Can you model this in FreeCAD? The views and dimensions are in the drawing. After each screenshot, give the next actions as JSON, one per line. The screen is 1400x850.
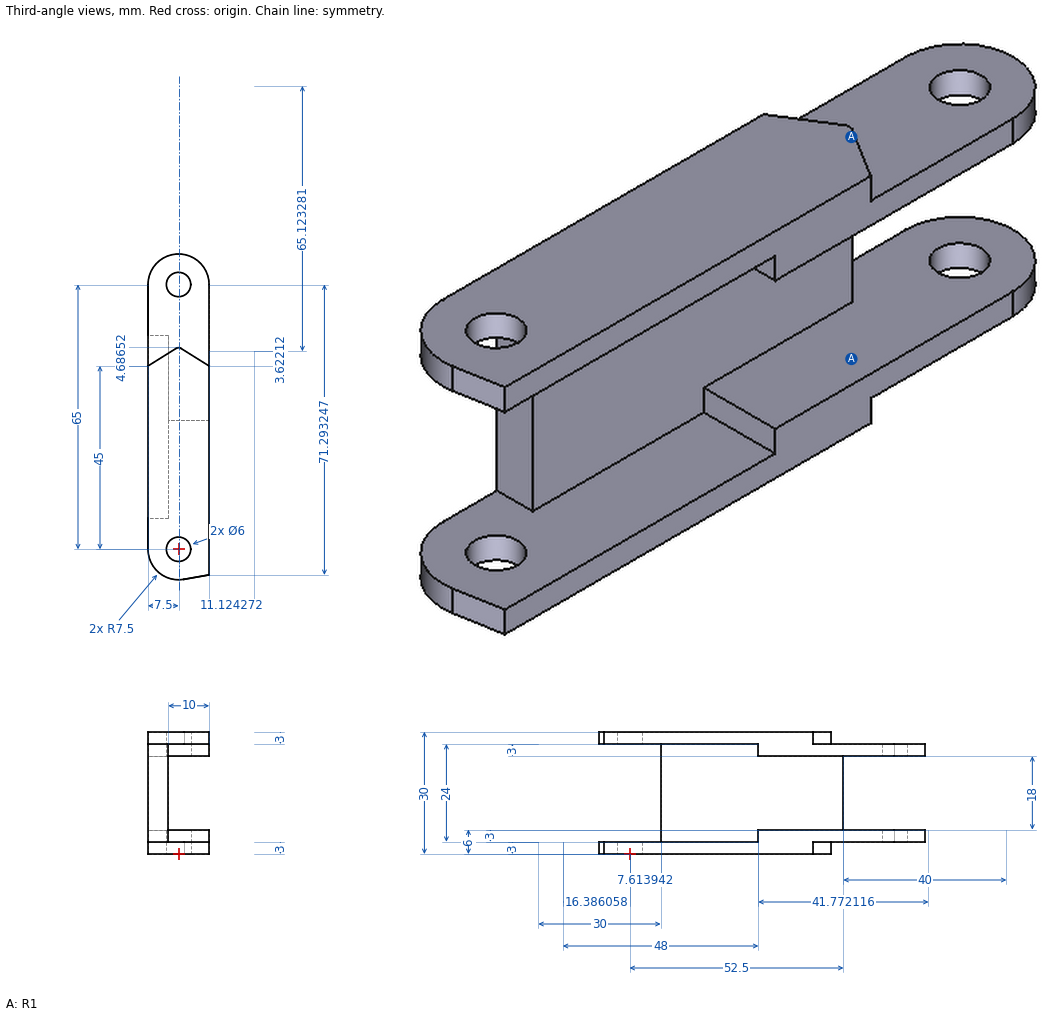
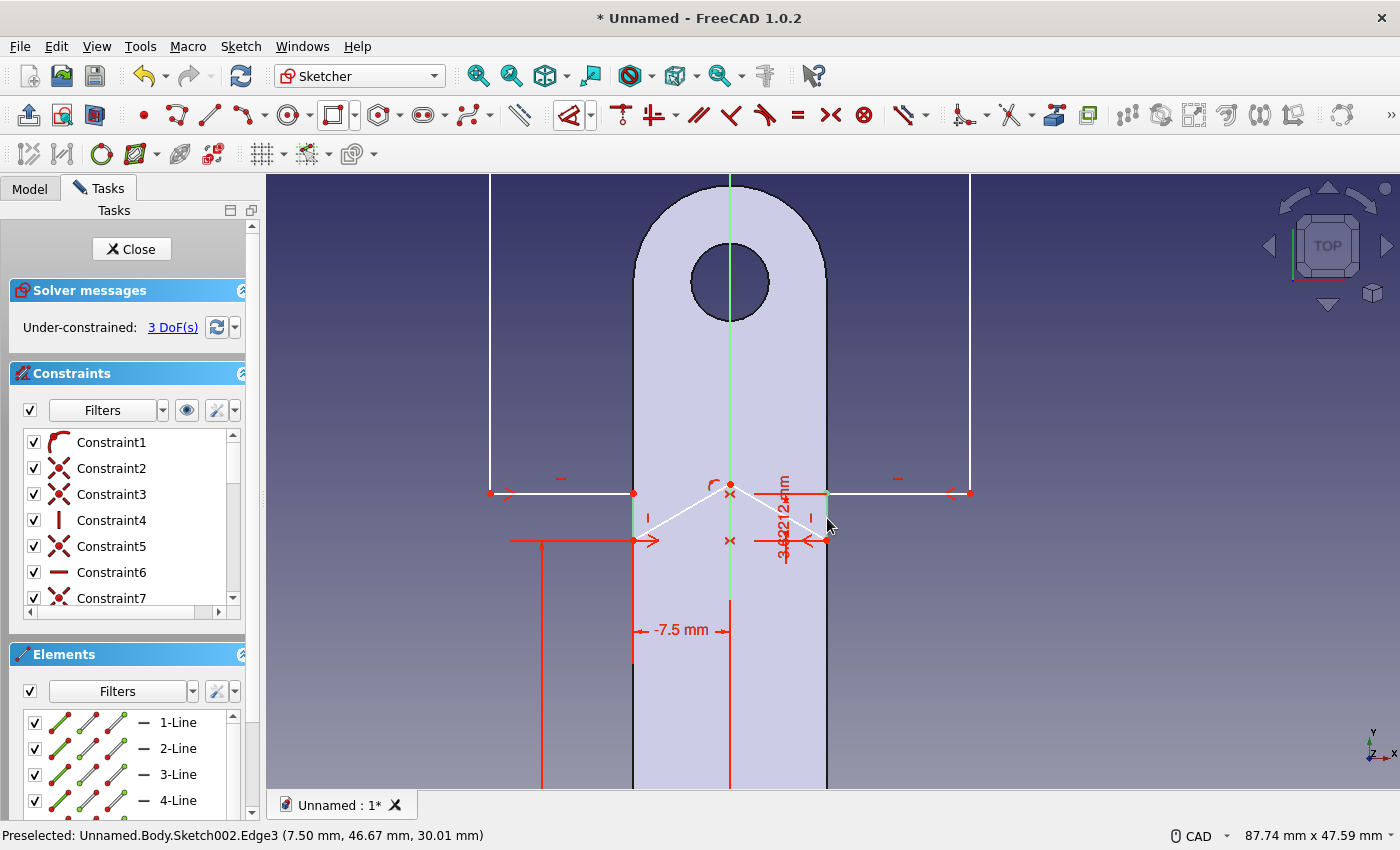
{"action": "left_click", "coordinate": [662, 524]}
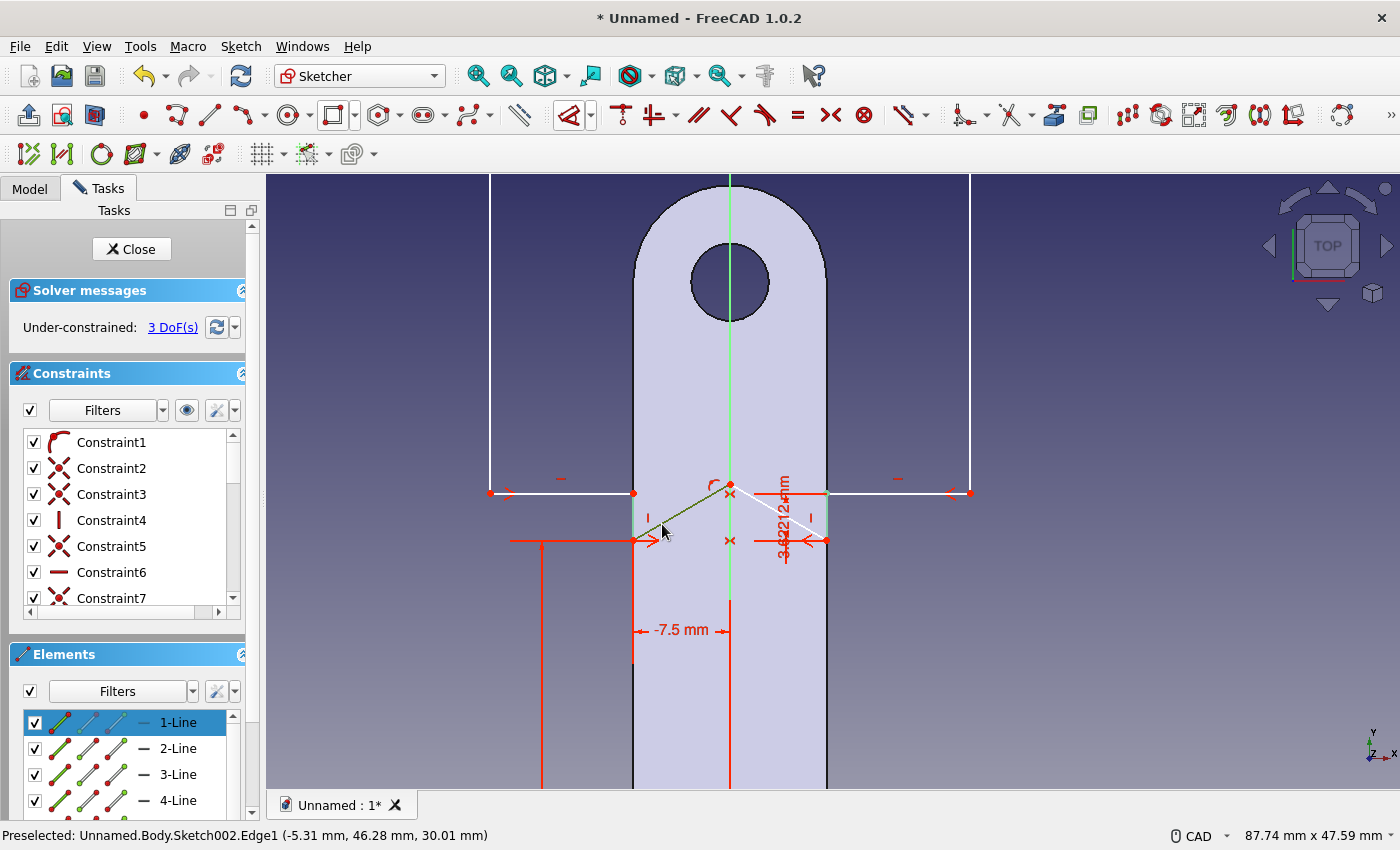
{"action": "key", "text": "i"}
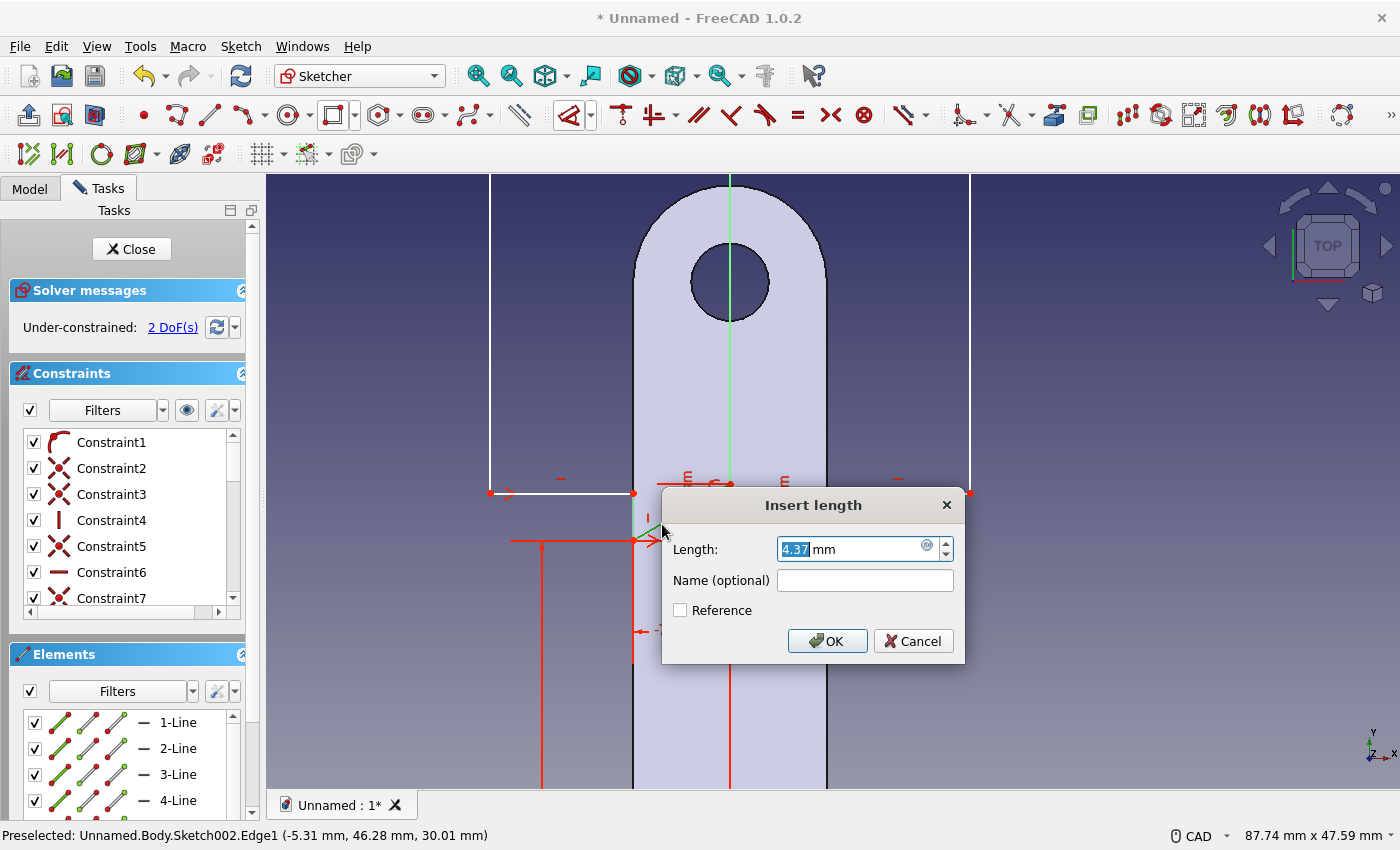
{"action": "type", "text": "4.68652"}
{"action": "key", "text": "Return"}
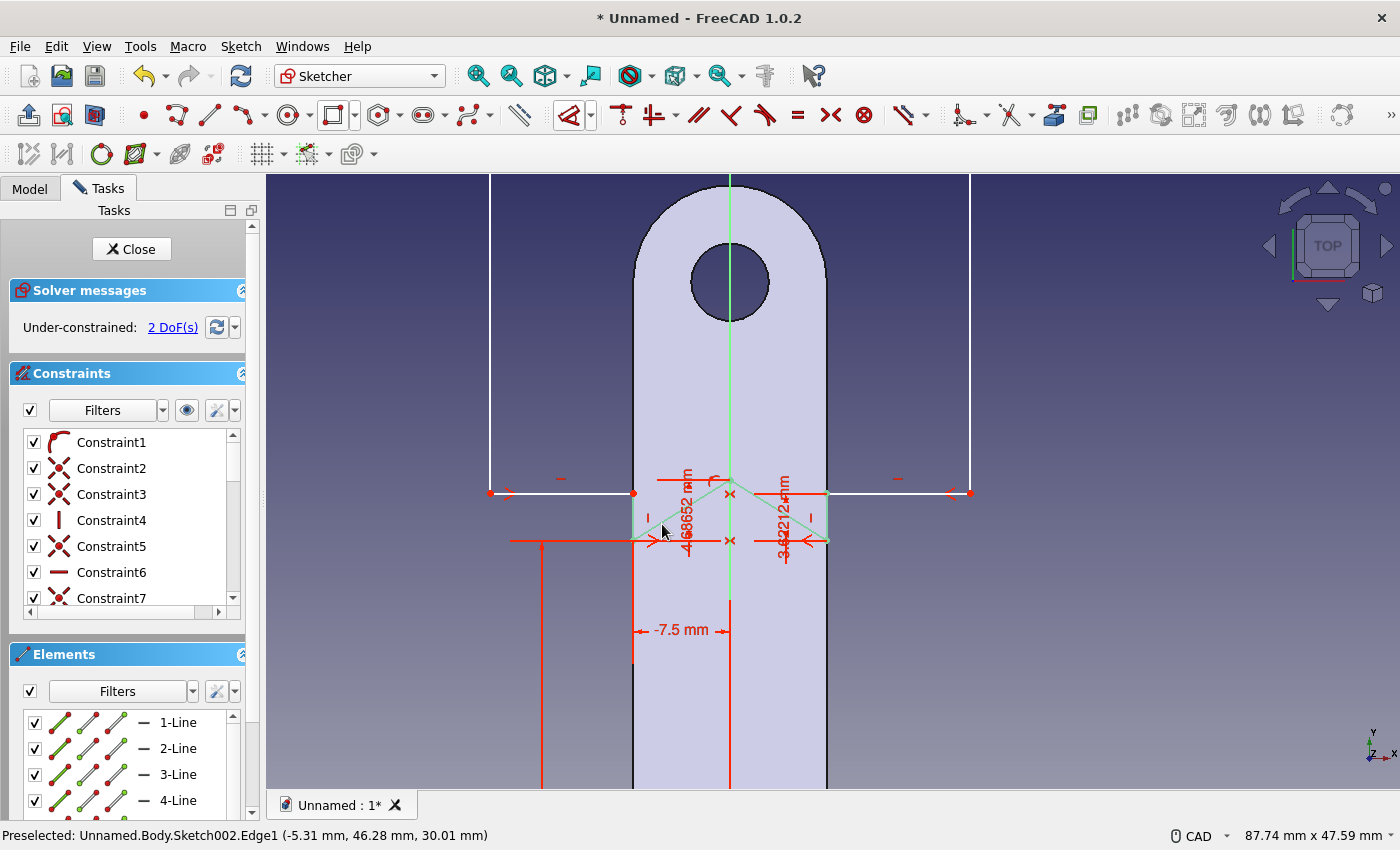
{"action": "scroll", "coordinate": [776, 512], "scroll_direction": "down", "scroll_amount": 7}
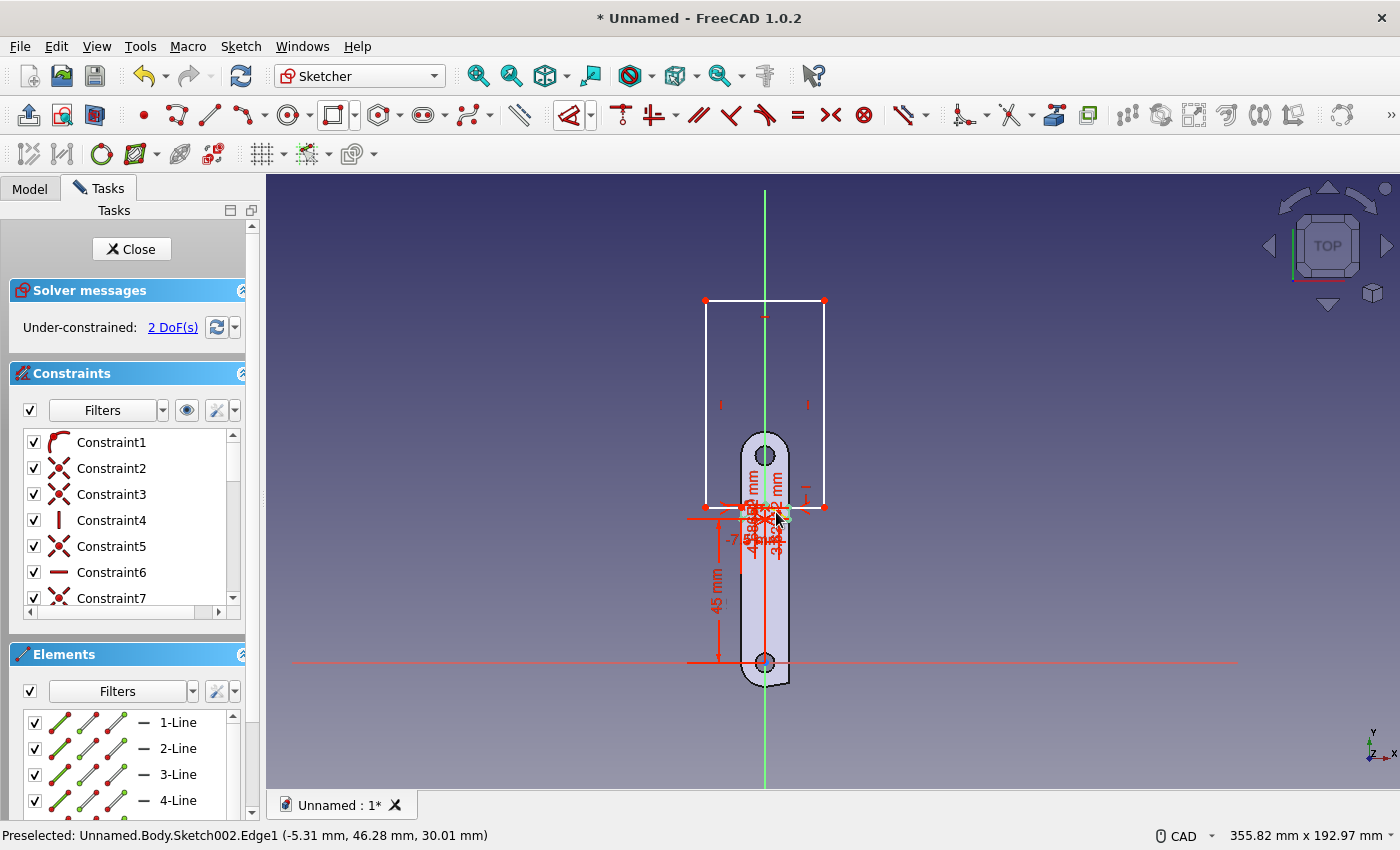
{"action": "scroll", "coordinate": [799, 508], "scroll_direction": "up", "scroll_amount": 2}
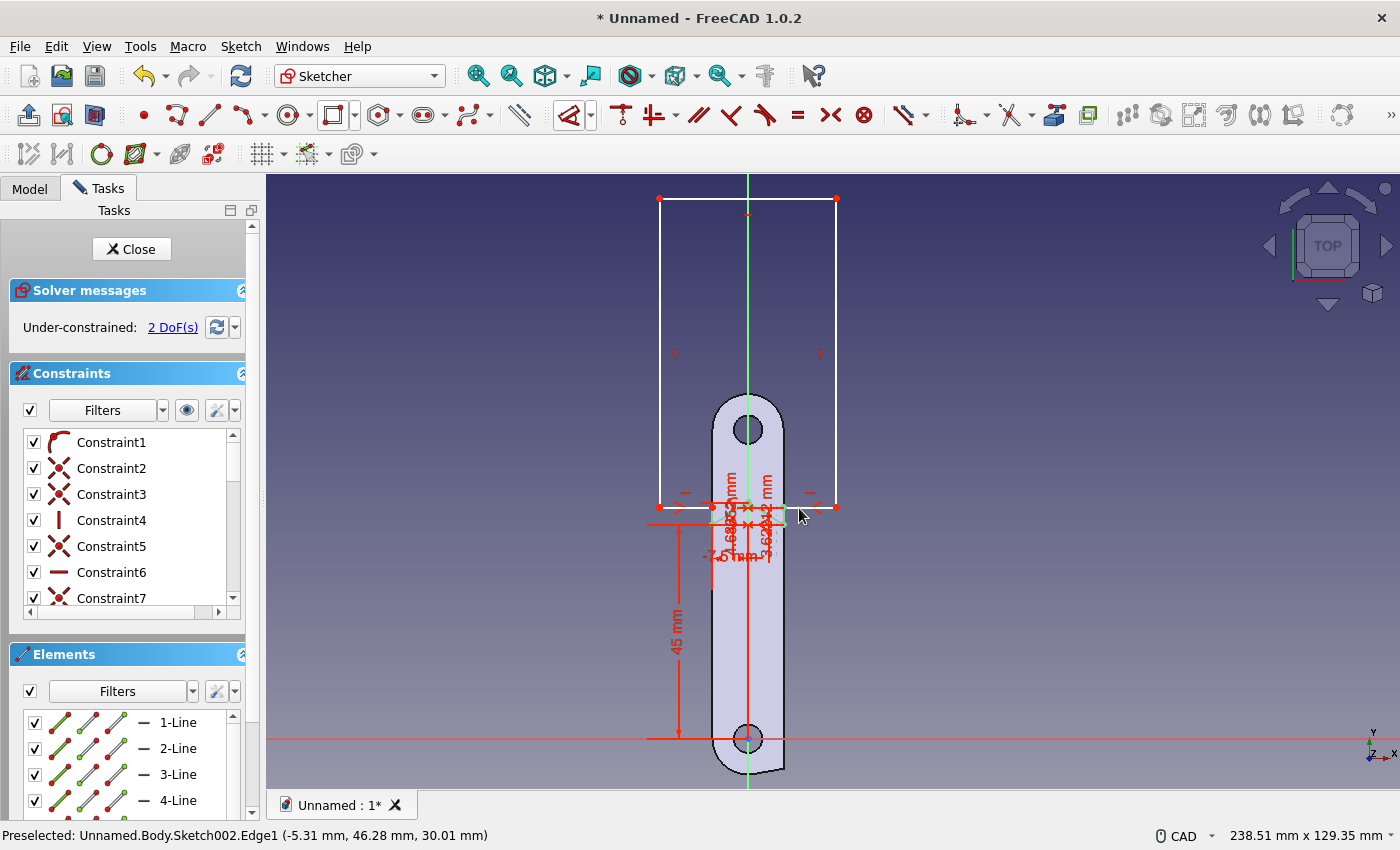
{"action": "left_click", "coordinate": [800, 508]}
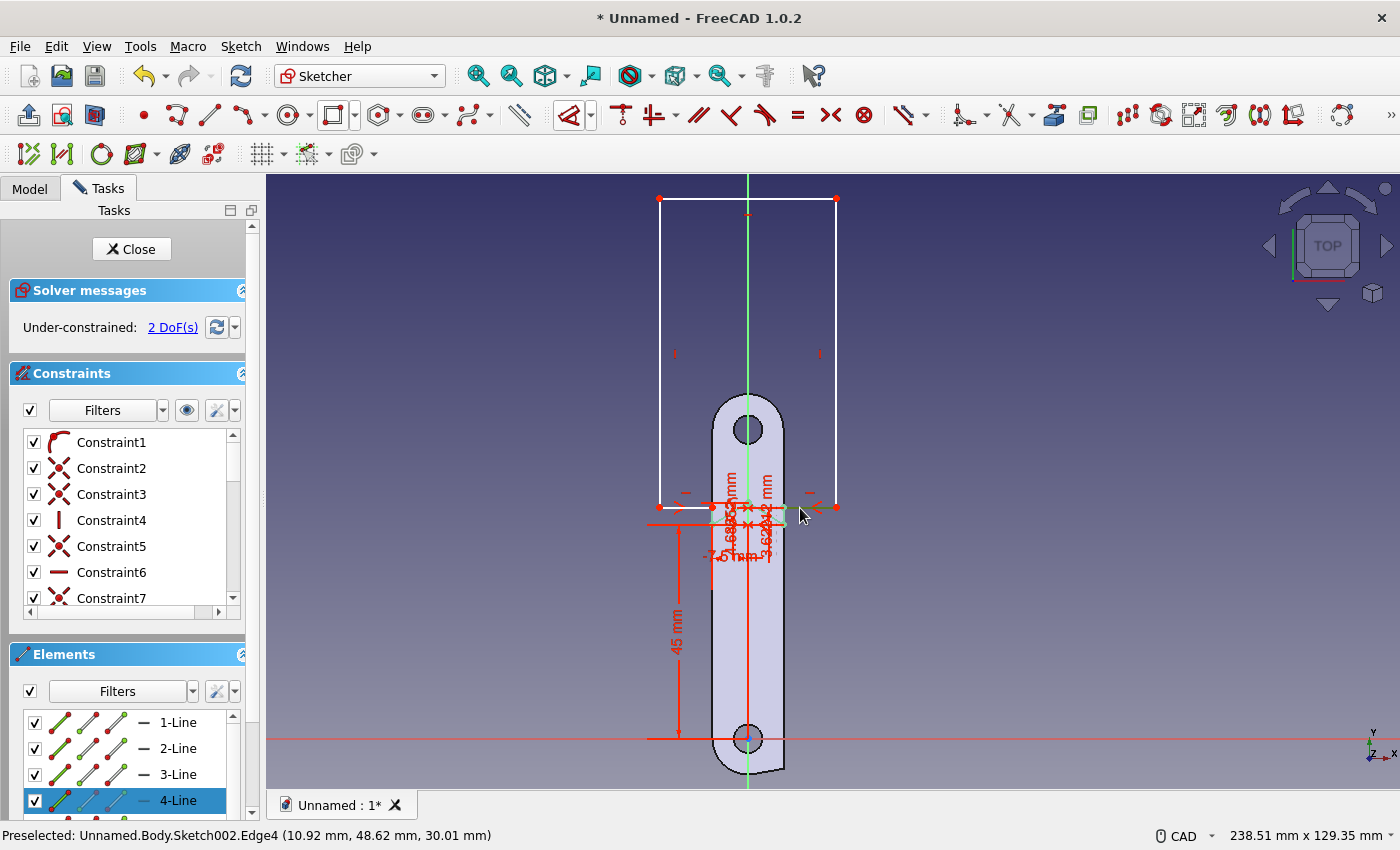
{"action": "key", "text": "l"}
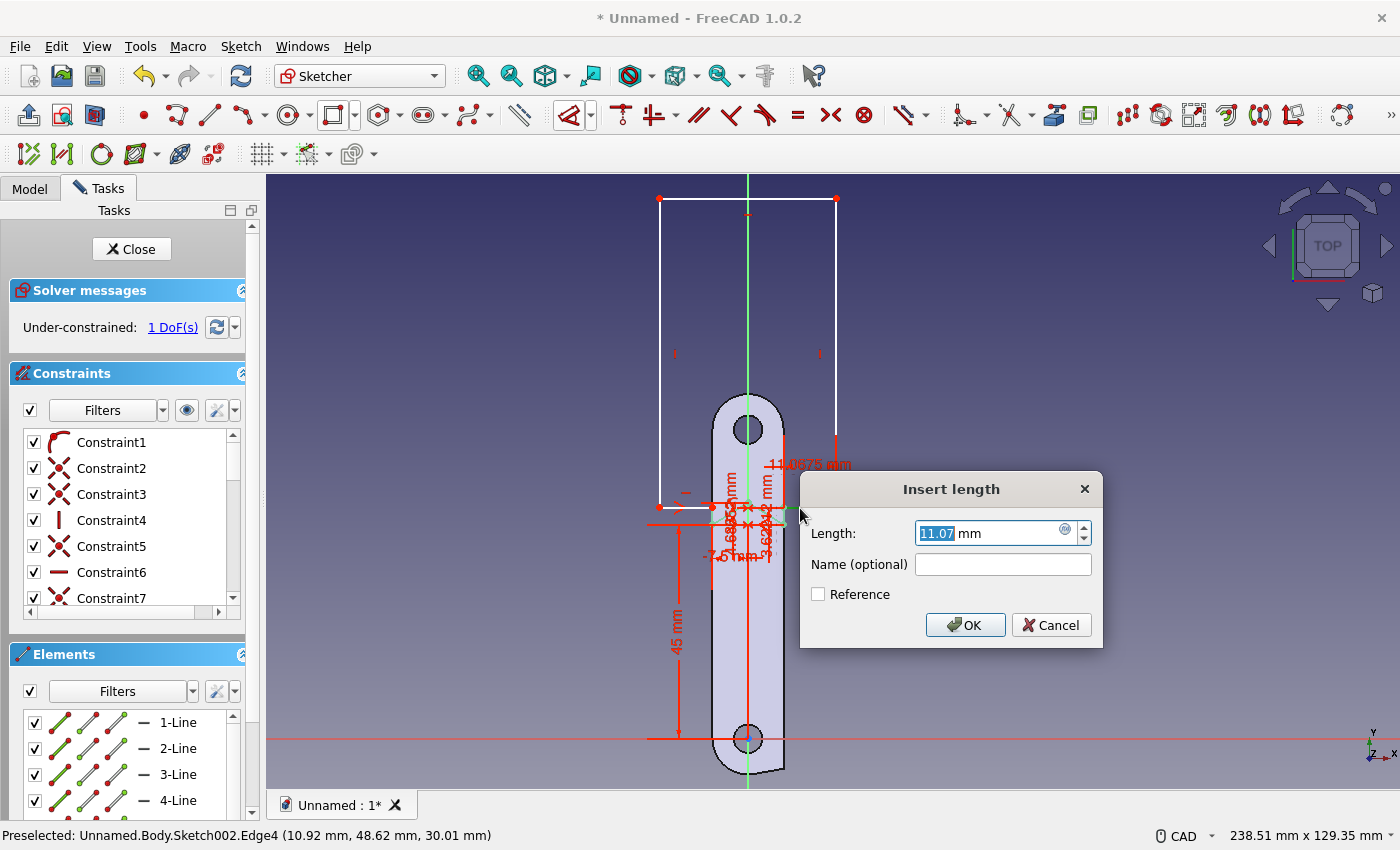
{"action": "type", "text": "11.124272"}
{"action": "key", "text": "Return"}